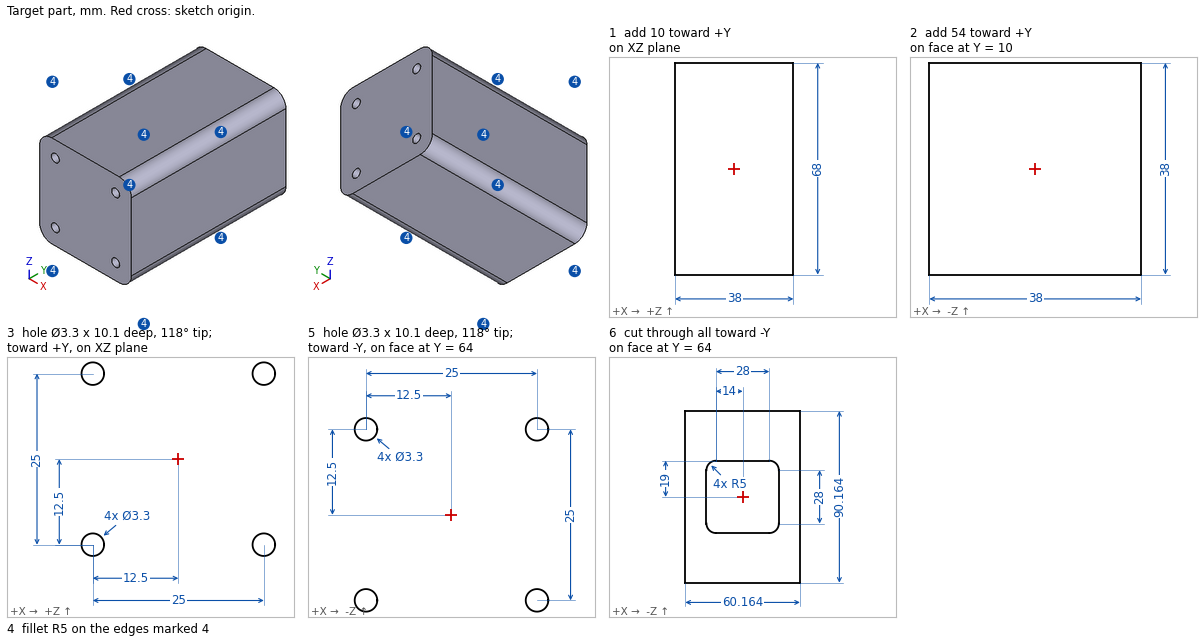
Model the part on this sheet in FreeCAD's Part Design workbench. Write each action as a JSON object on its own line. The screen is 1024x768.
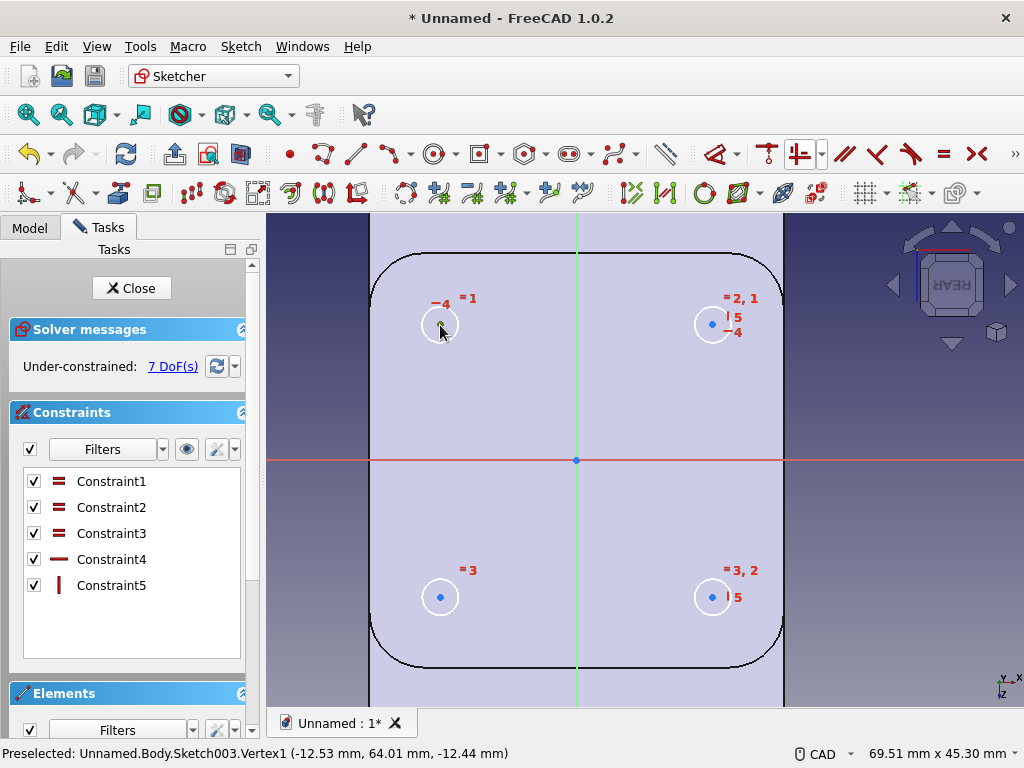
{"action": "left_click", "coordinate": [440, 597]}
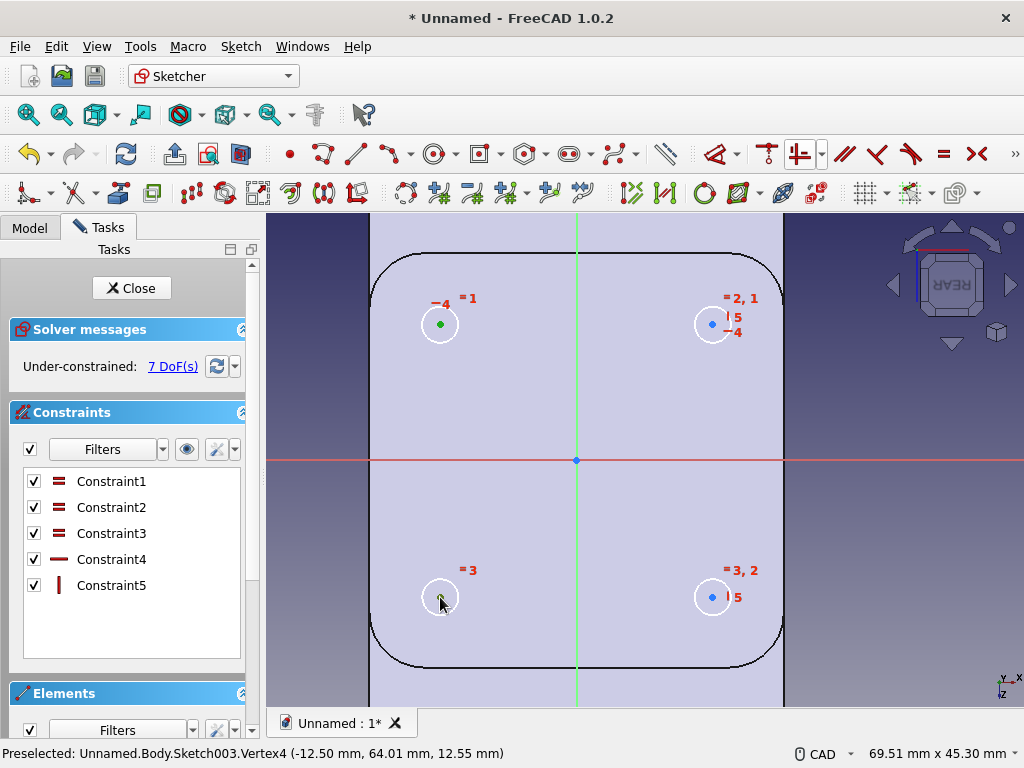
{"action": "left_click", "coordinate": [822, 154]}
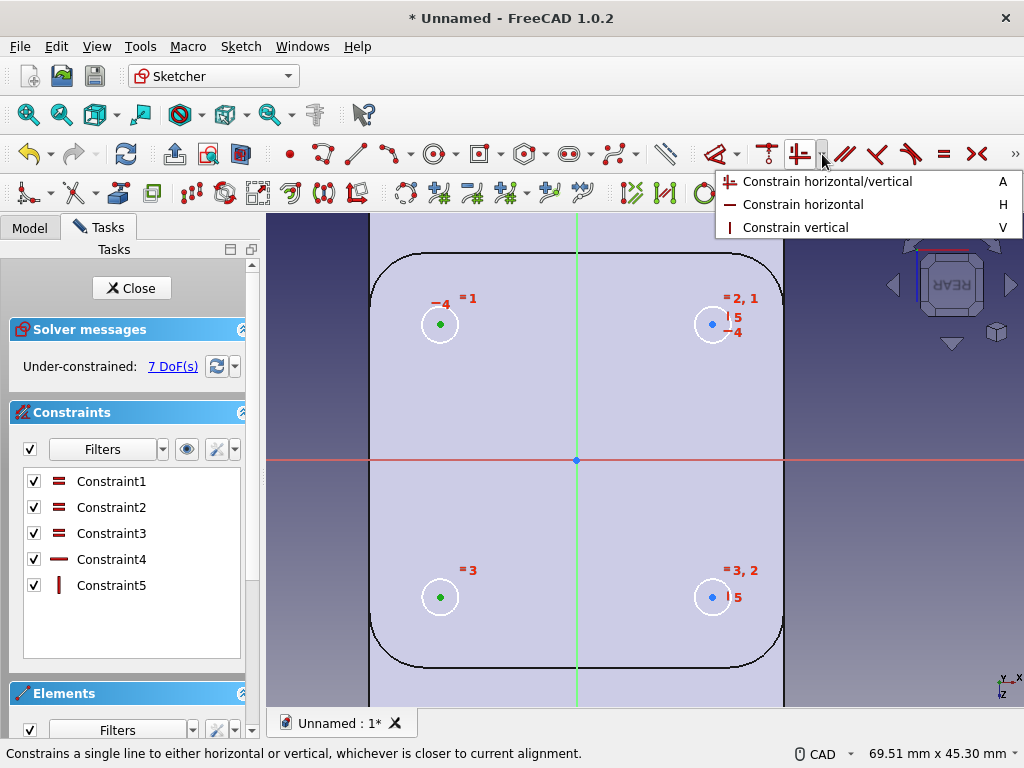
{"action": "left_click", "coordinate": [869, 228]}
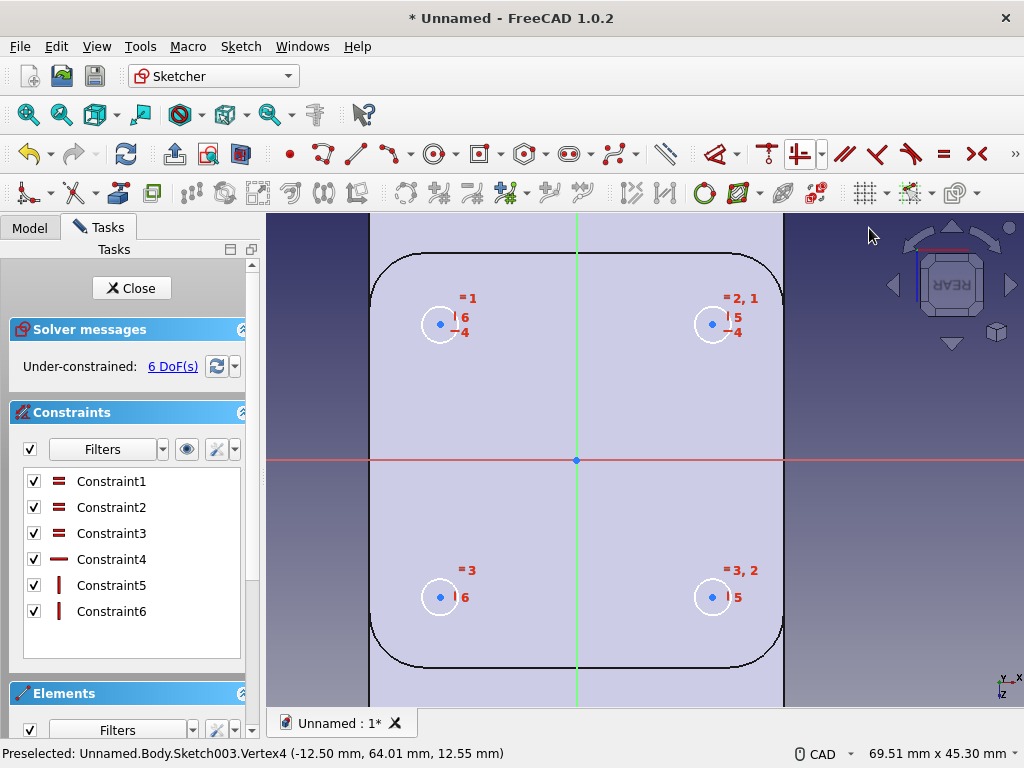
{"action": "left_click", "coordinate": [713, 597]}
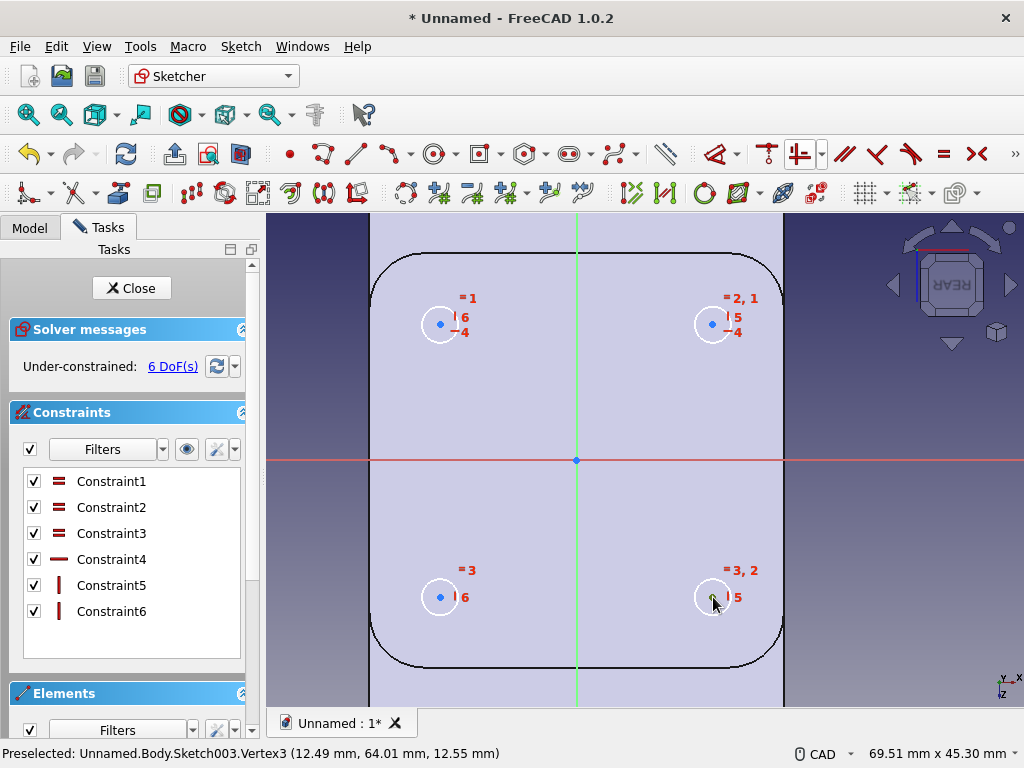
{"action": "left_click", "coordinate": [440, 597]}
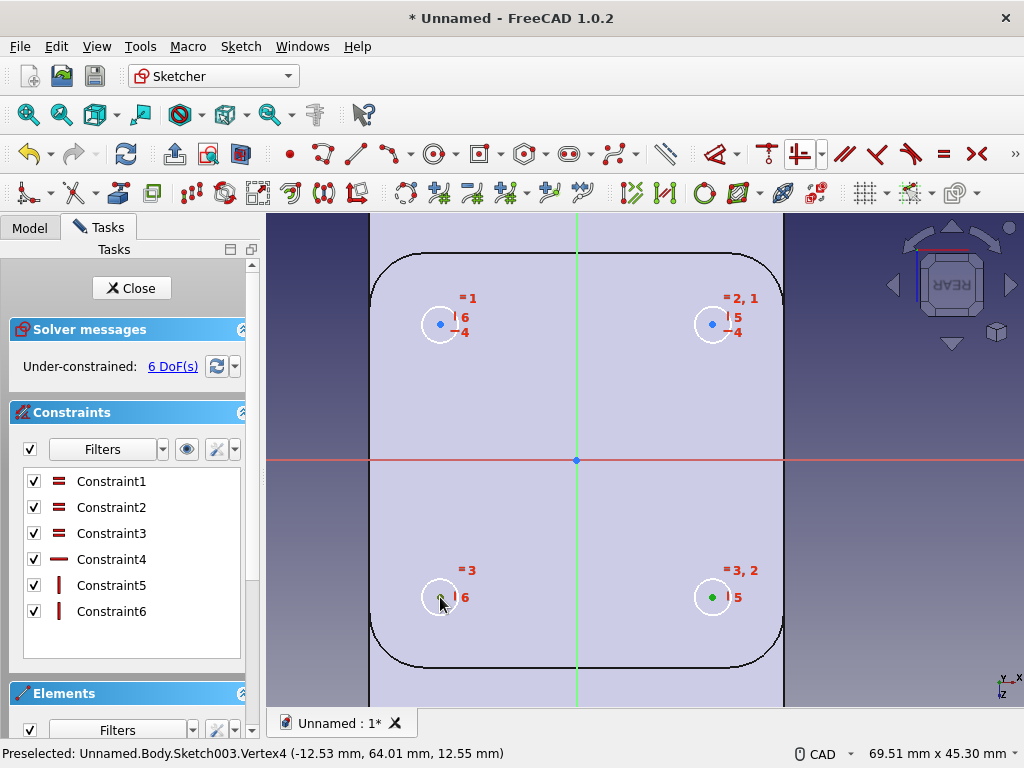
{"action": "left_click", "coordinate": [822, 154]}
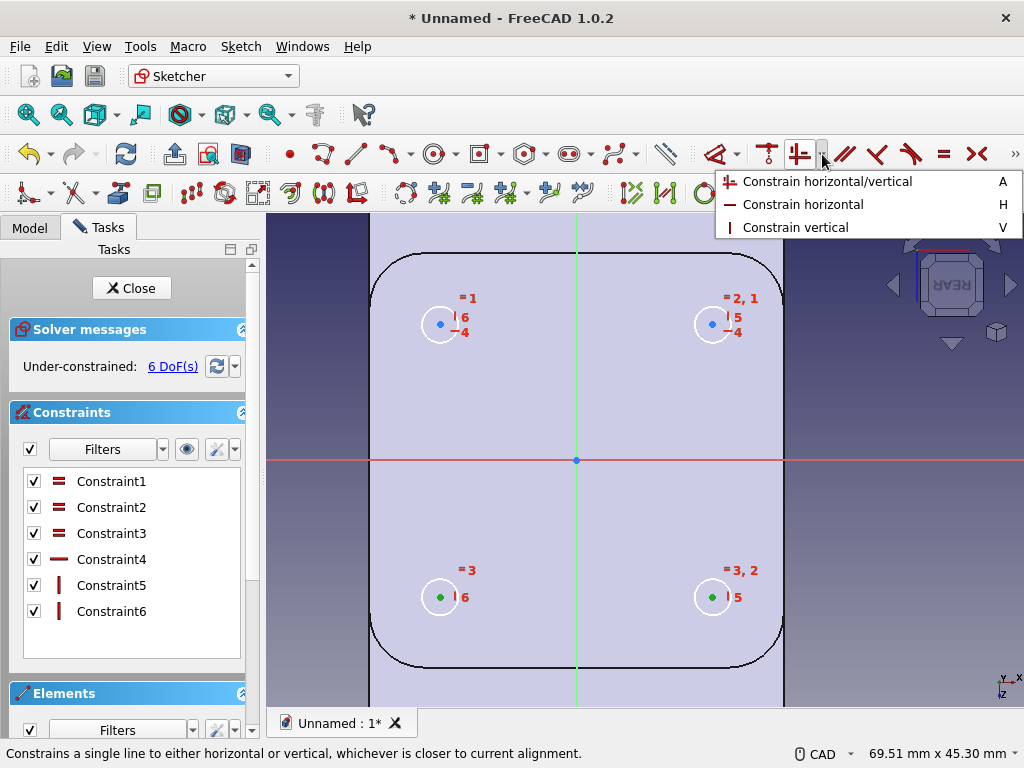
{"action": "left_click", "coordinate": [869, 204]}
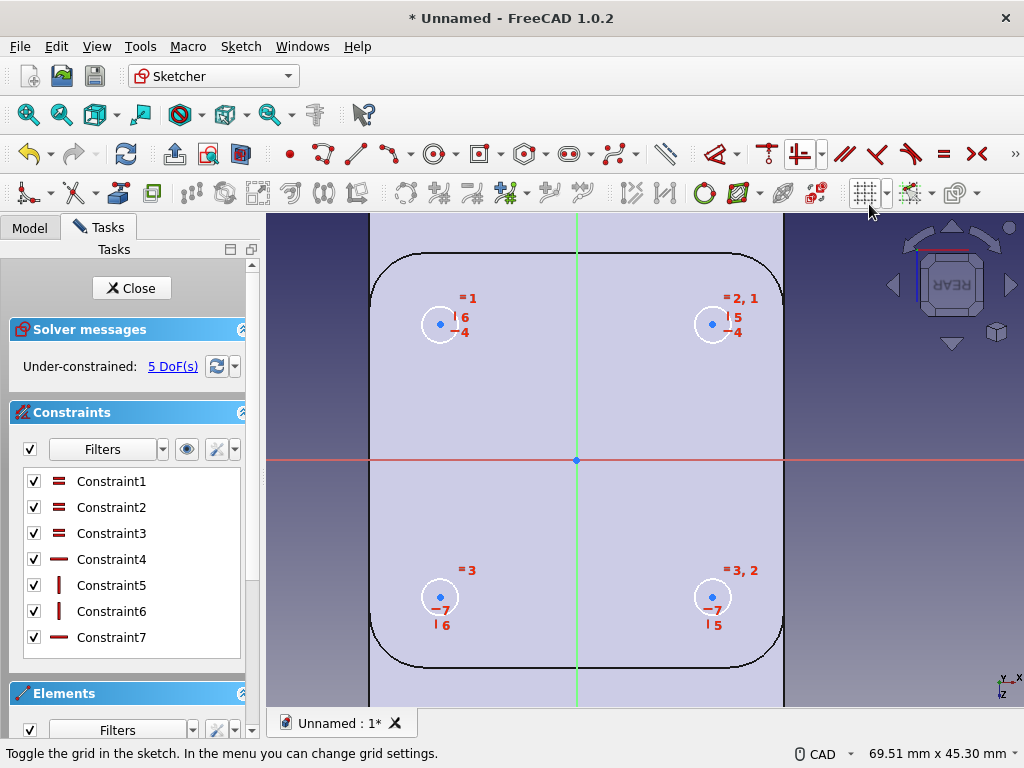
{"action": "left_click", "coordinate": [714, 154]}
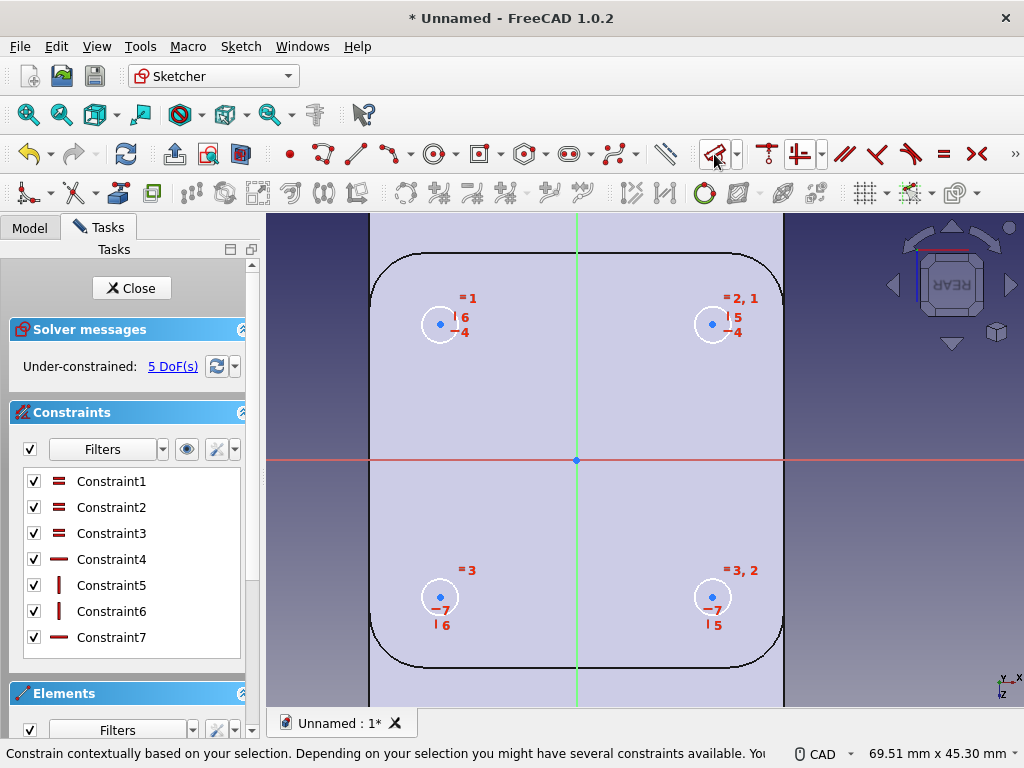
{"action": "left_click", "coordinate": [453, 312]}
{"action": "left_click", "coordinate": [476, 290]}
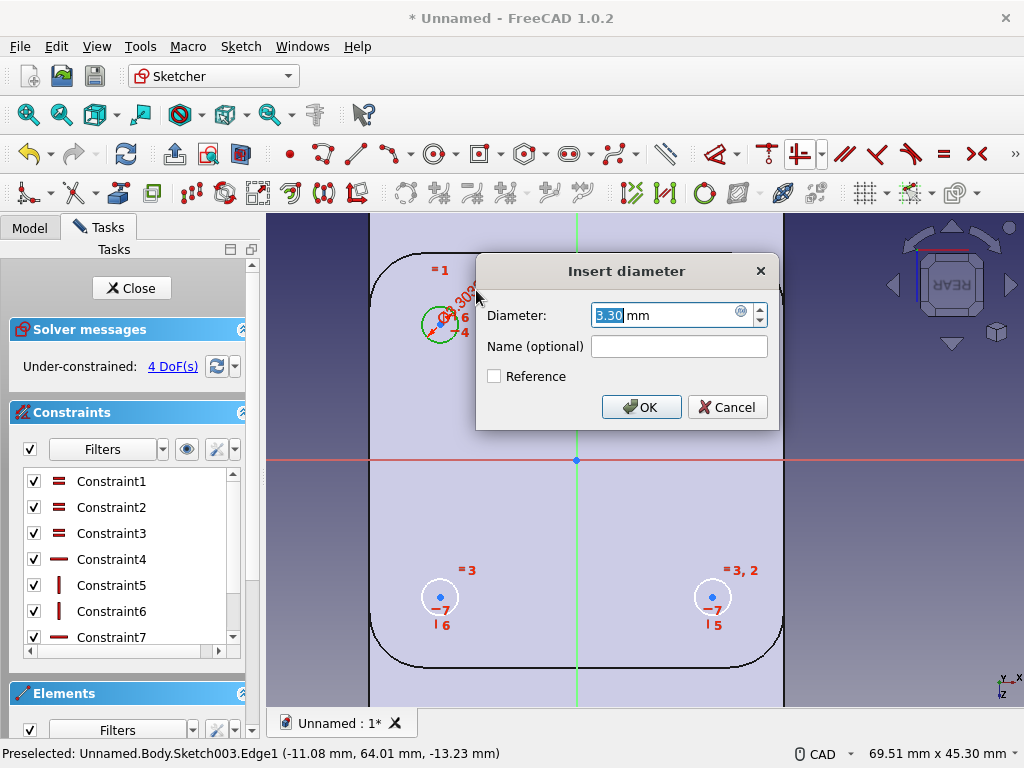
{"action": "type", "text": "3.3"}
{"action": "key", "text": "Return"}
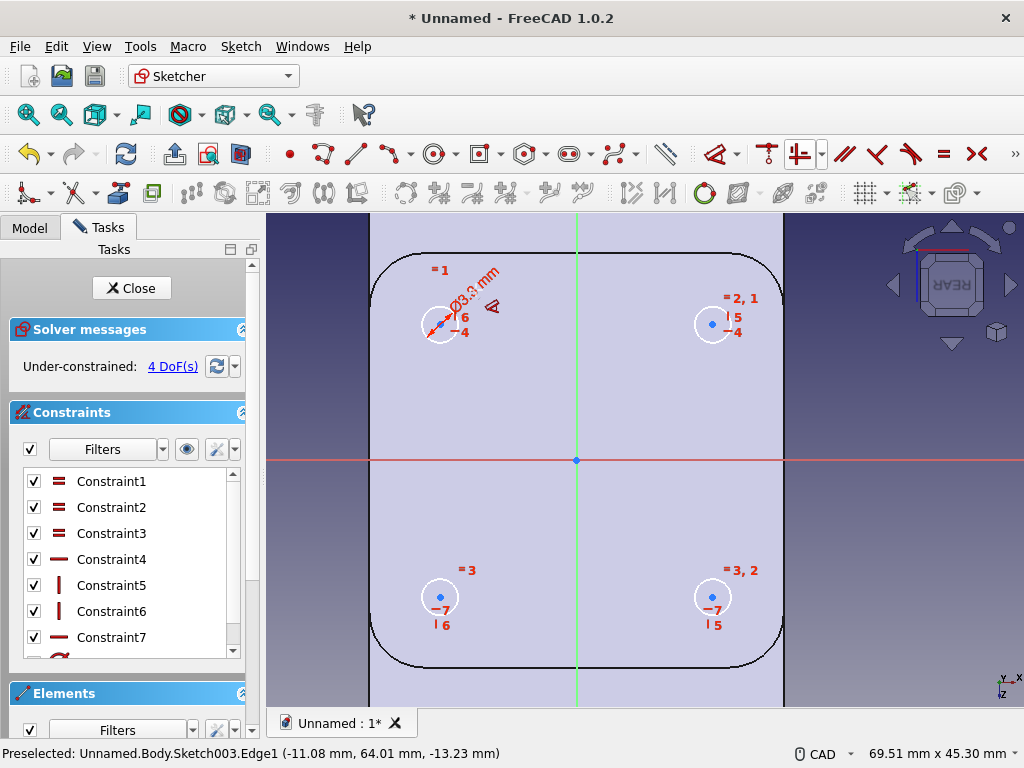
{"action": "left_click", "coordinate": [440, 325]}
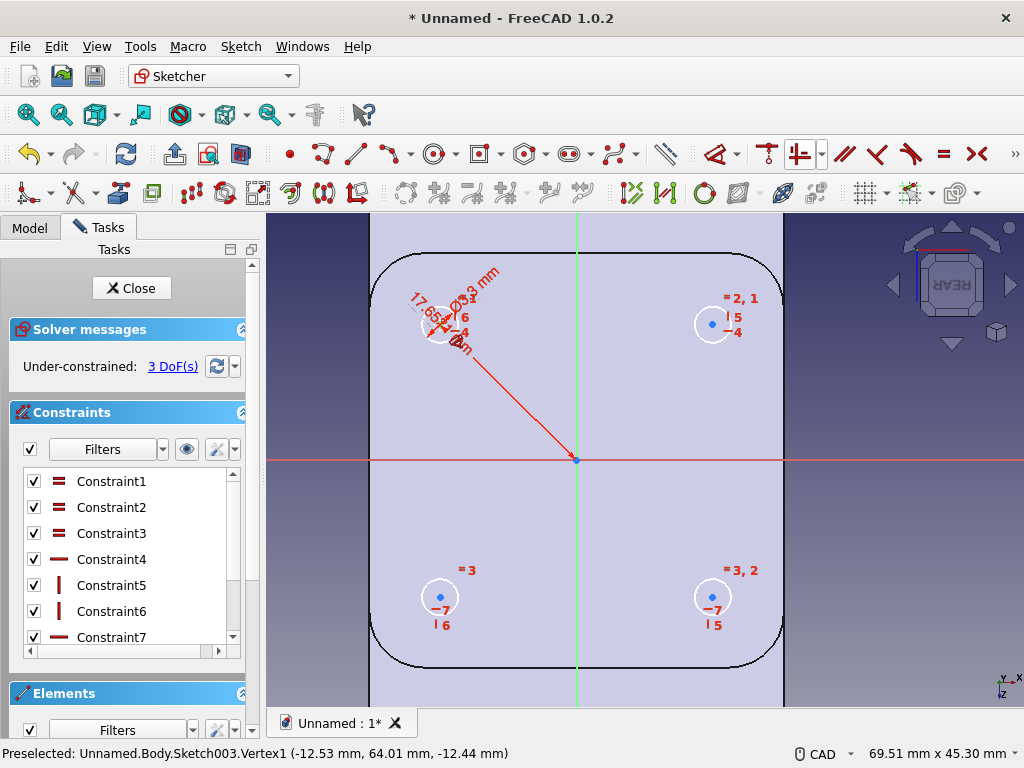
{"action": "left_click", "coordinate": [713, 325]}
{"action": "left_click", "coordinate": [639, 291]}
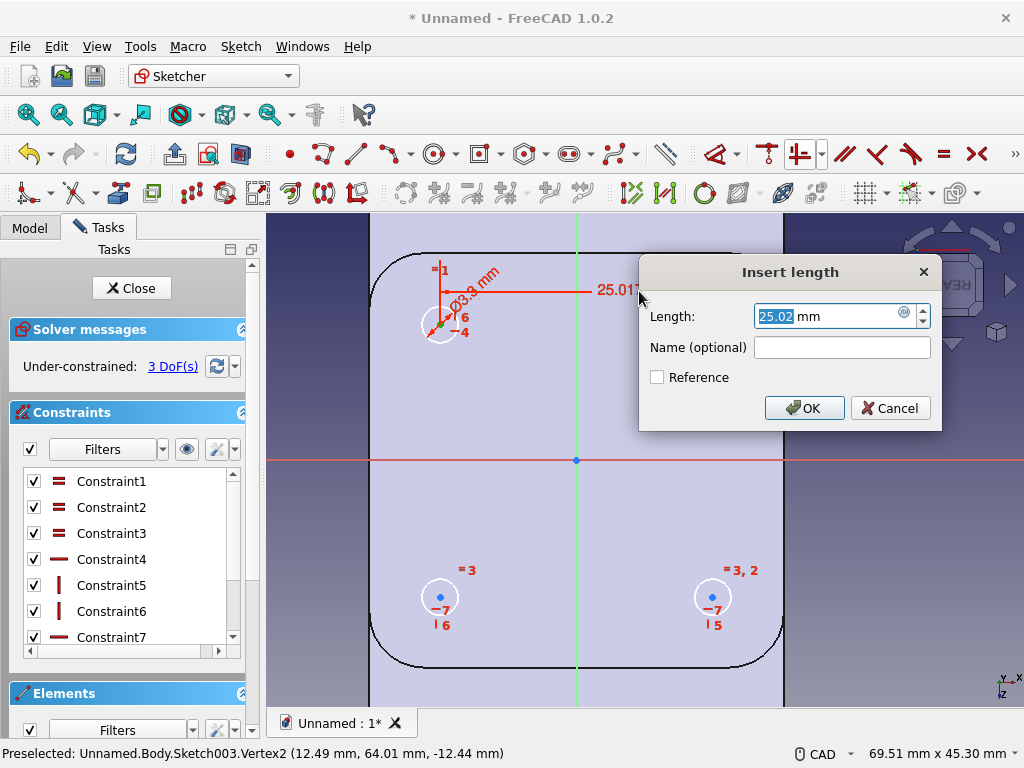
{"action": "type", "text": "25"}
{"action": "key", "text": "Return"}